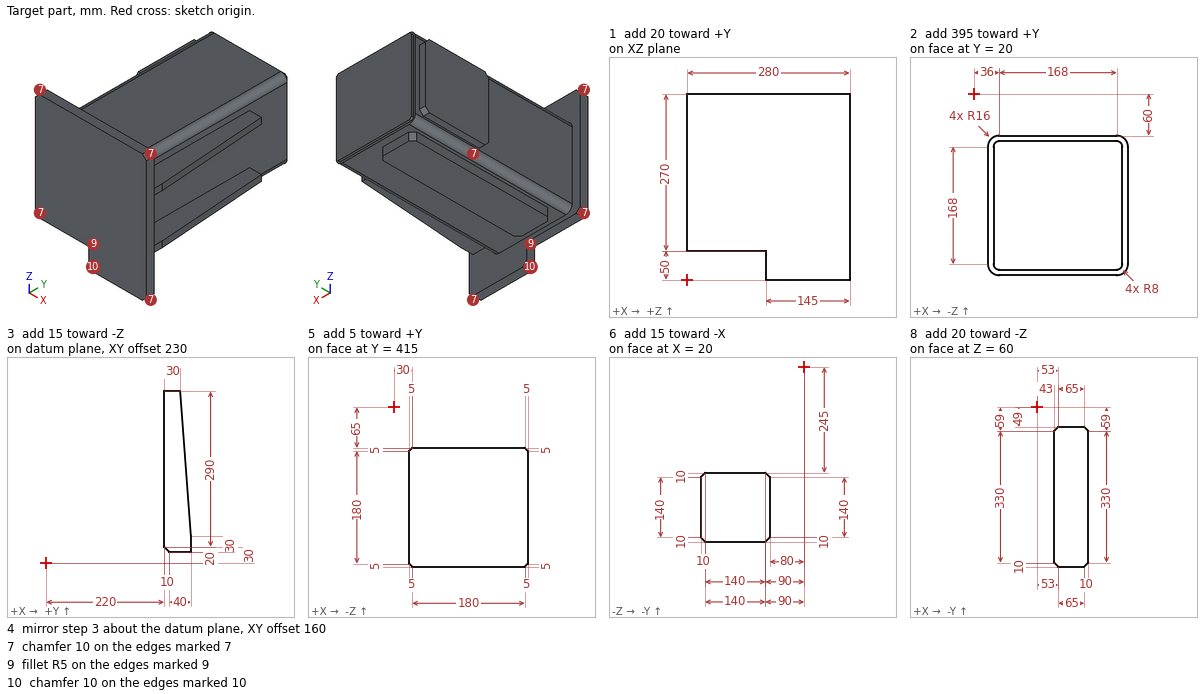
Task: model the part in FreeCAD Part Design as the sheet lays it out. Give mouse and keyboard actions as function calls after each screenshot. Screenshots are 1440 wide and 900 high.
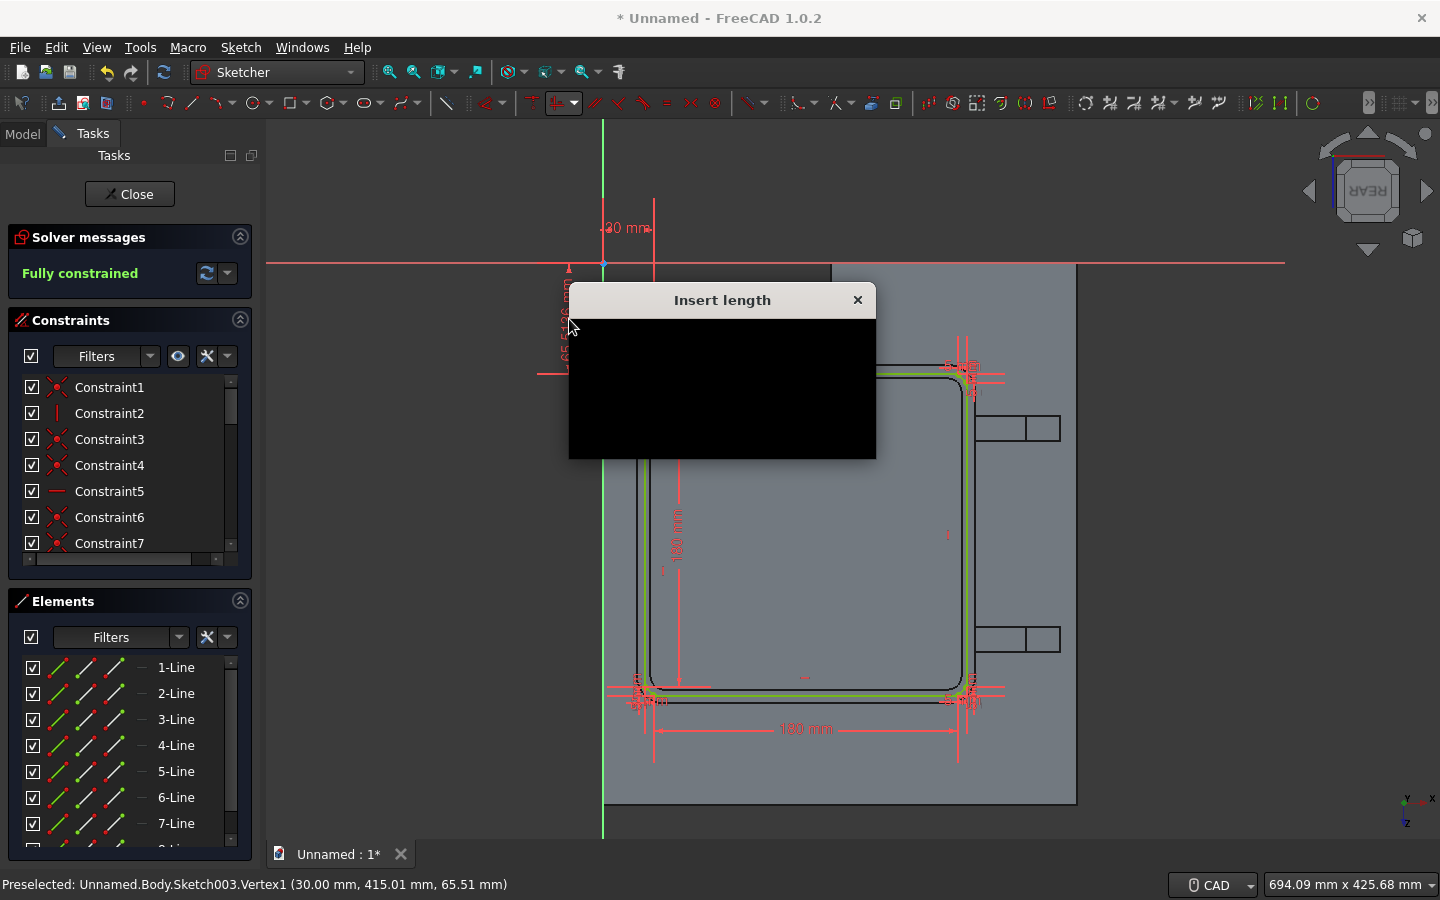
text(65)
key(Return)
key(Escape)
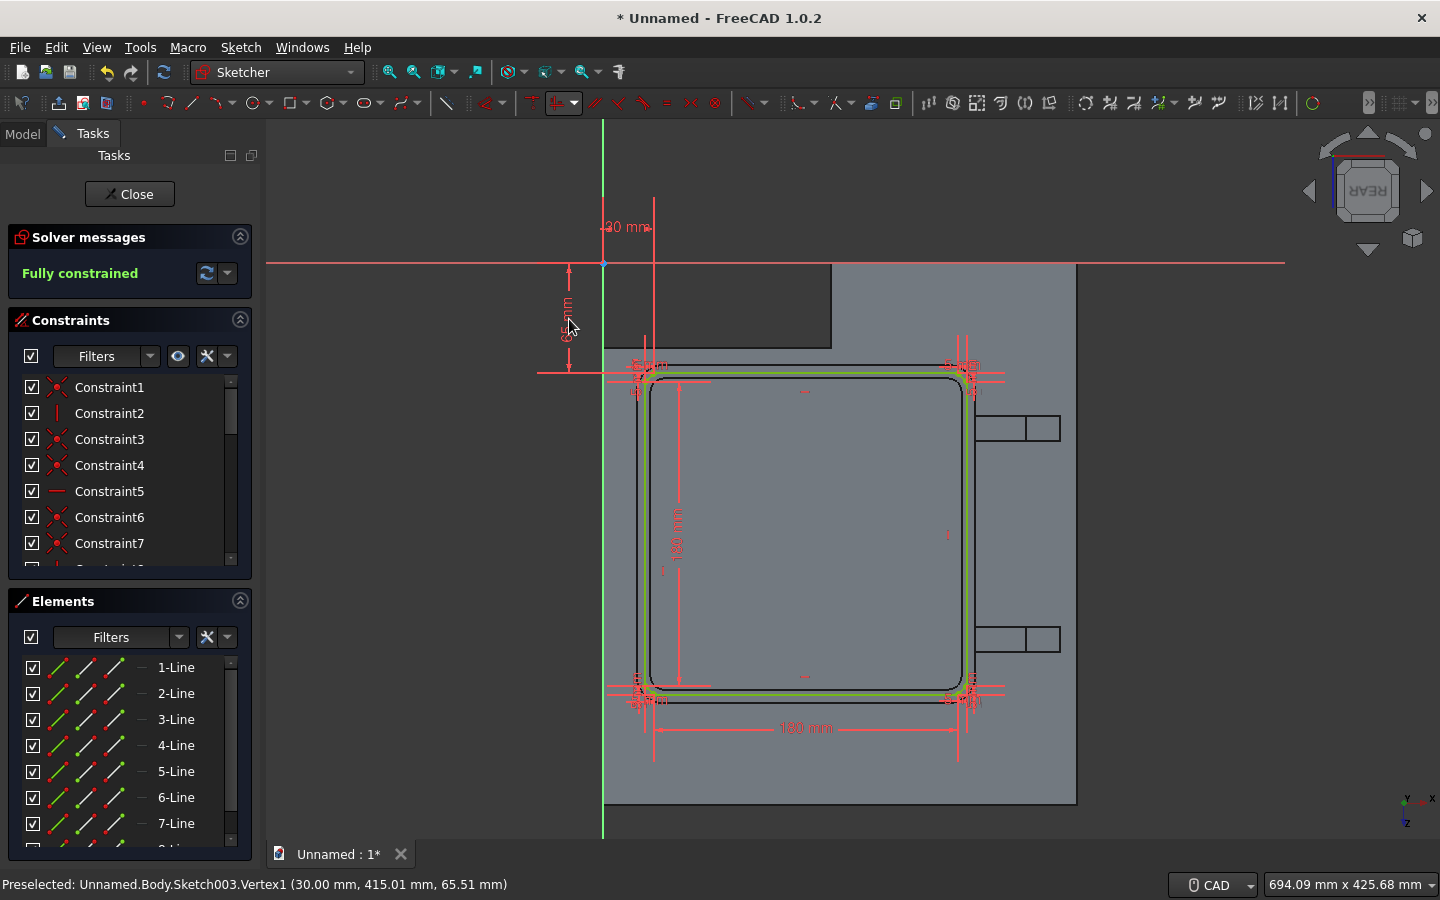
click(130, 194)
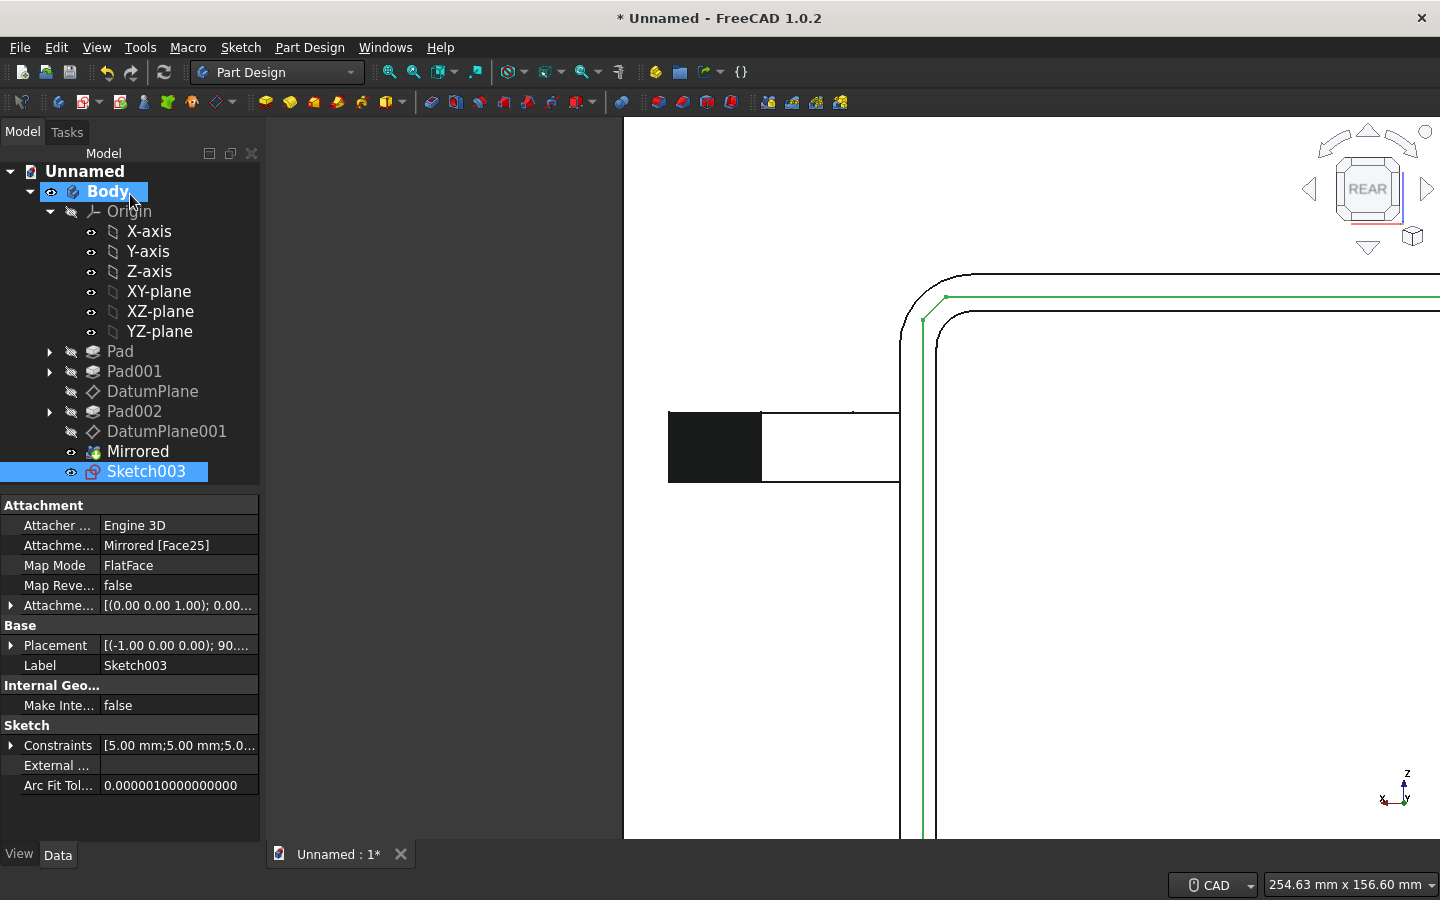
click(266, 102)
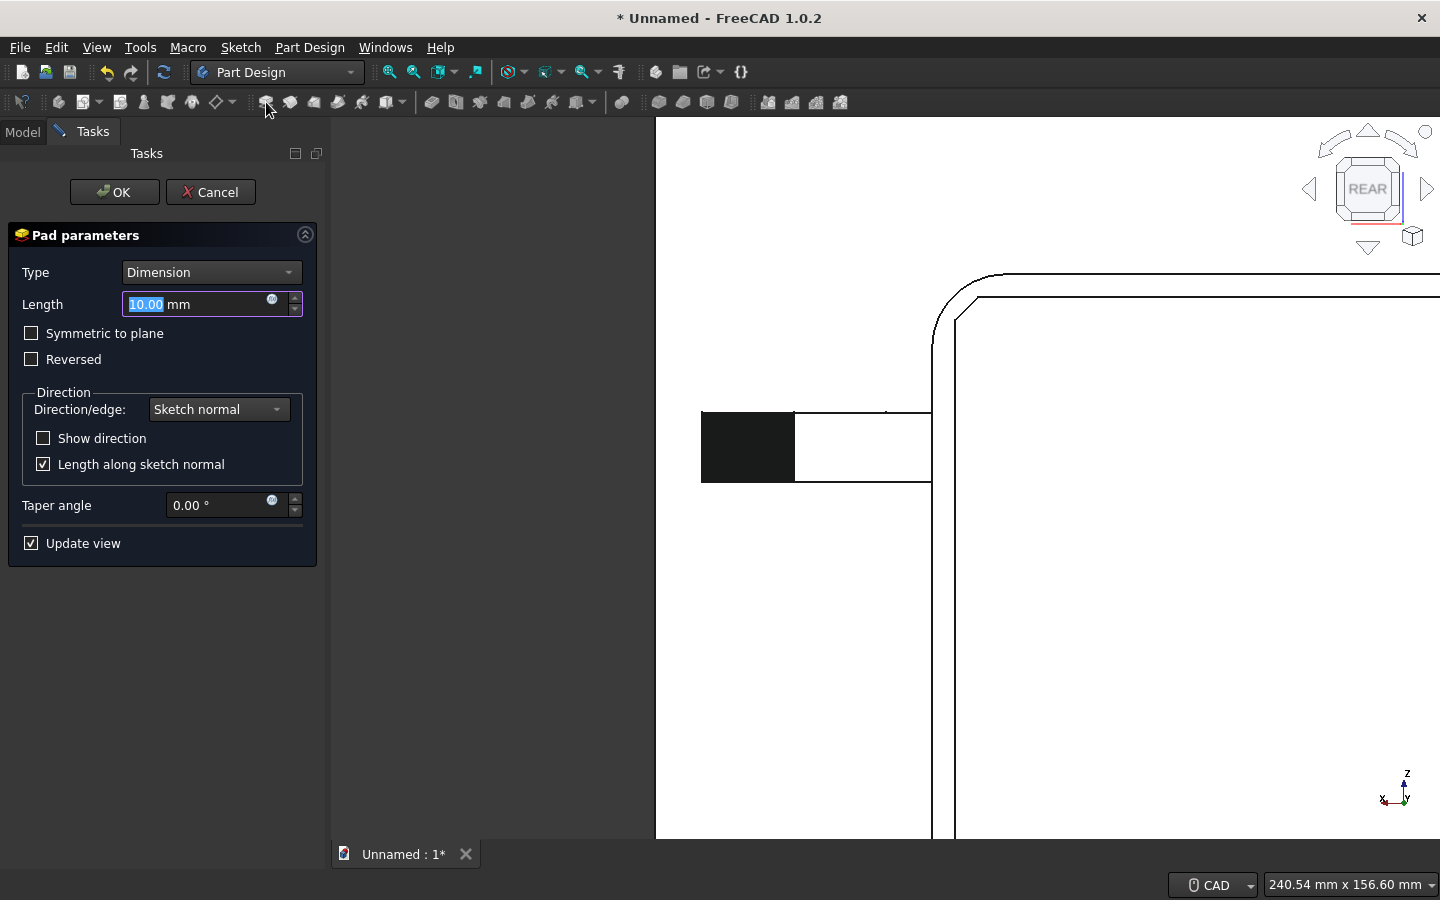
text(5)
key(Tab)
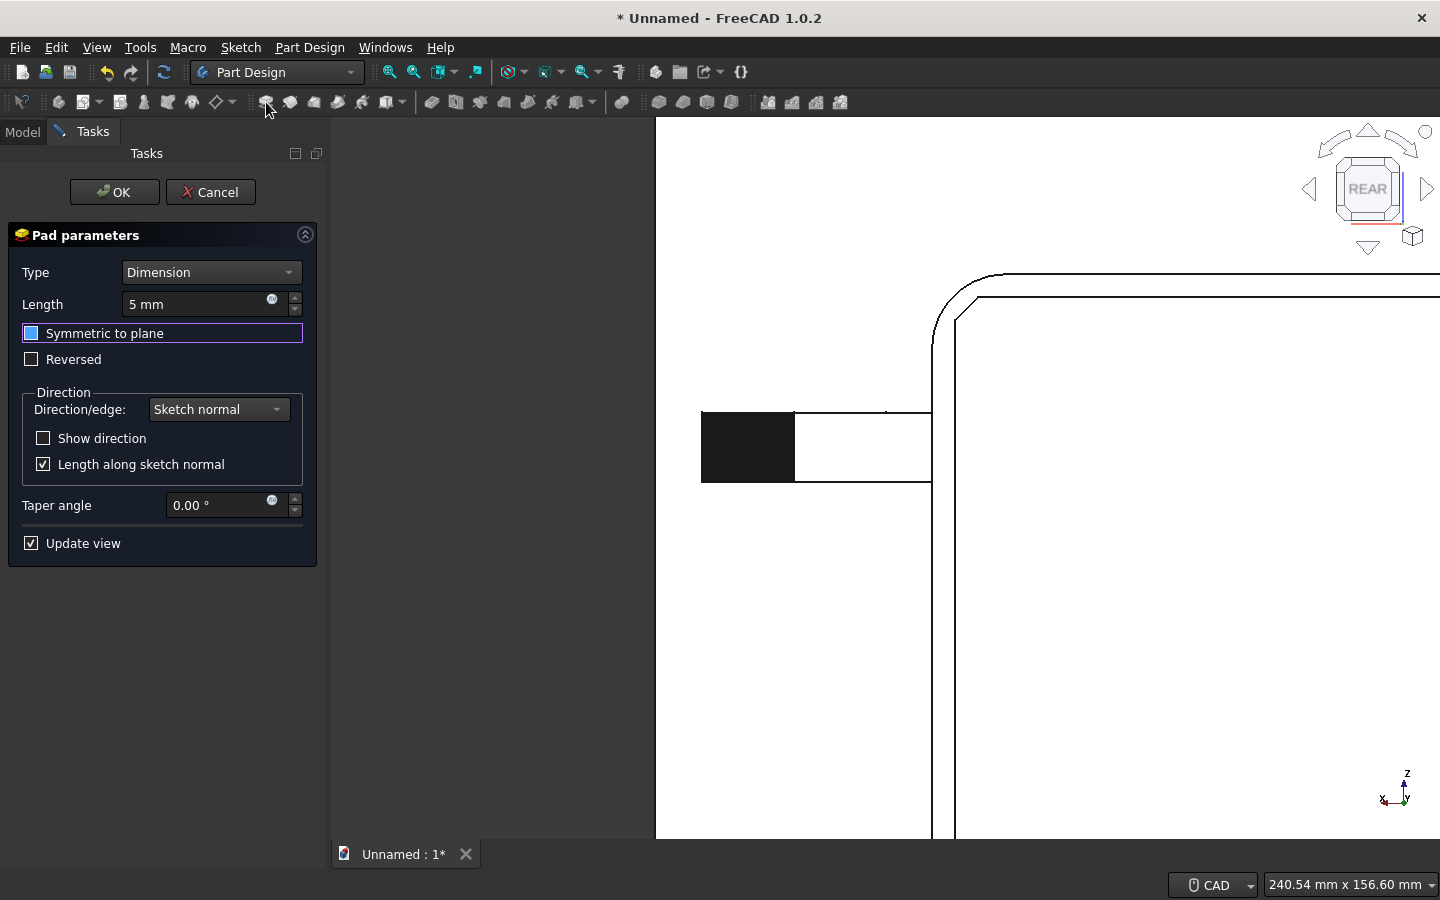
click(115, 192)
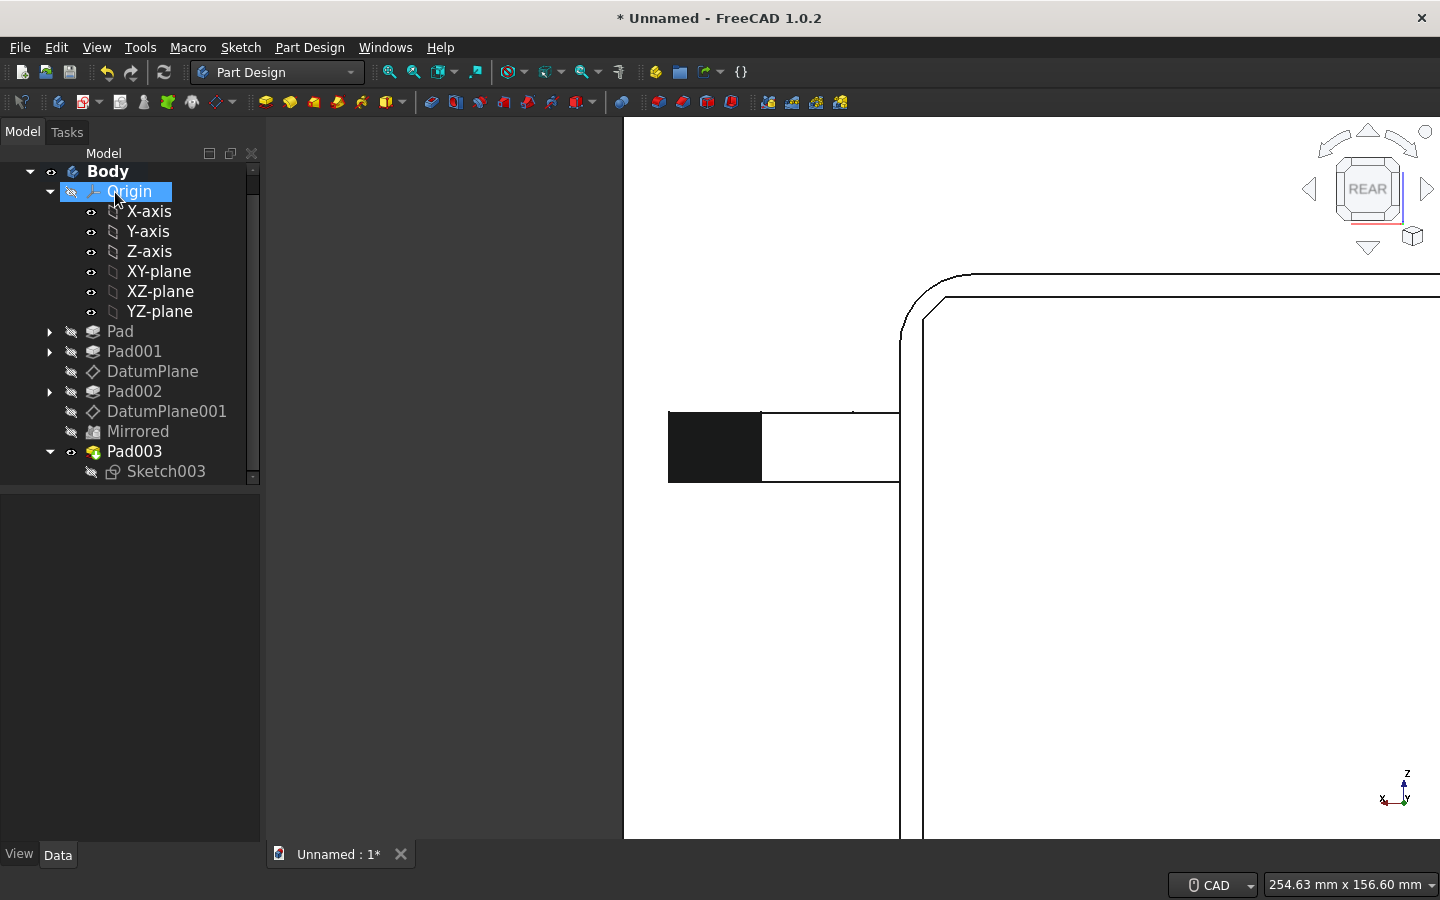
key(v)
key(f)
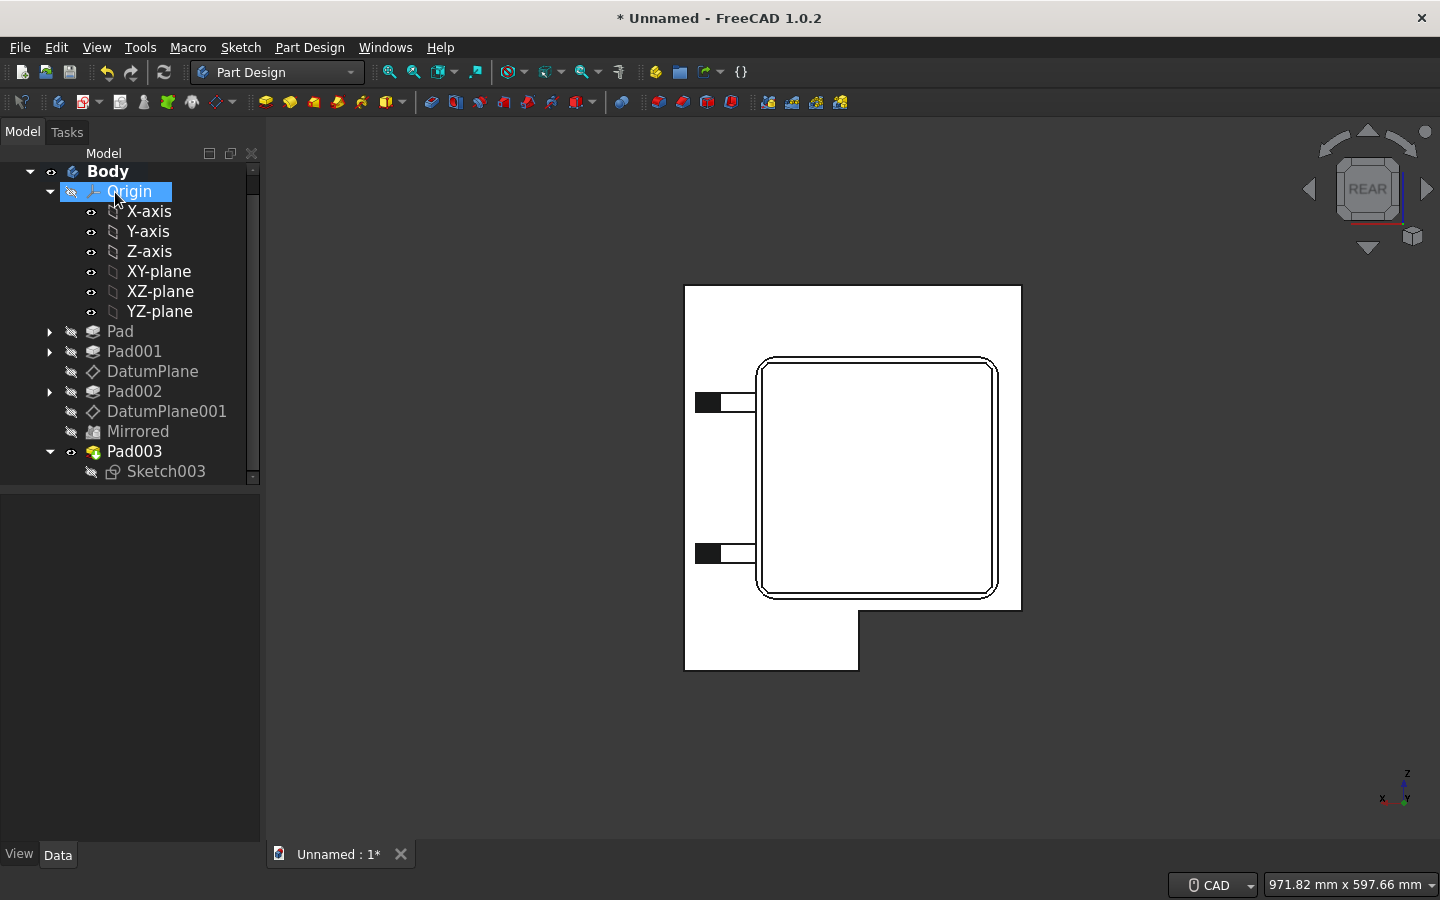
key(6)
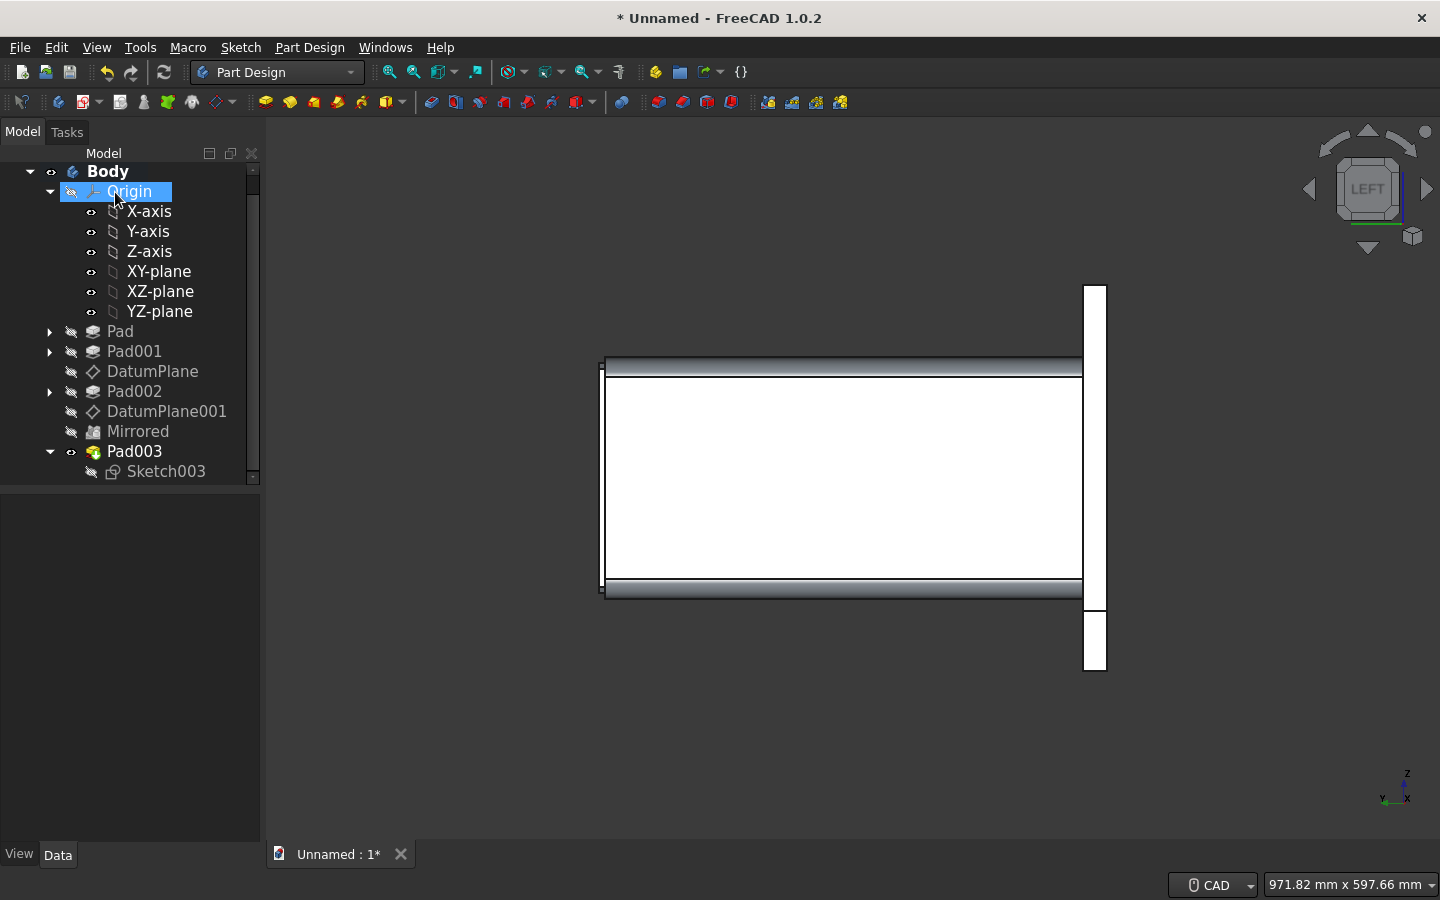
click(776, 477)